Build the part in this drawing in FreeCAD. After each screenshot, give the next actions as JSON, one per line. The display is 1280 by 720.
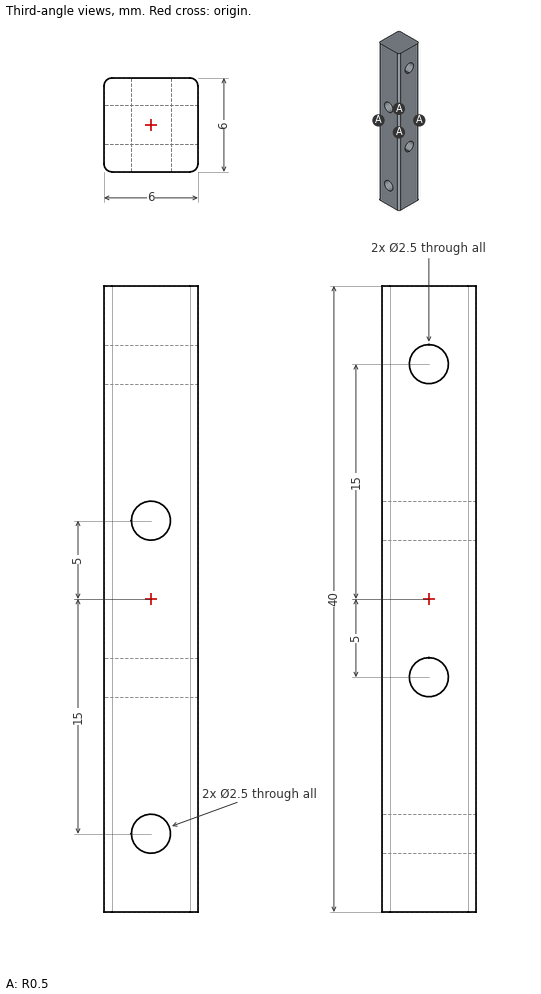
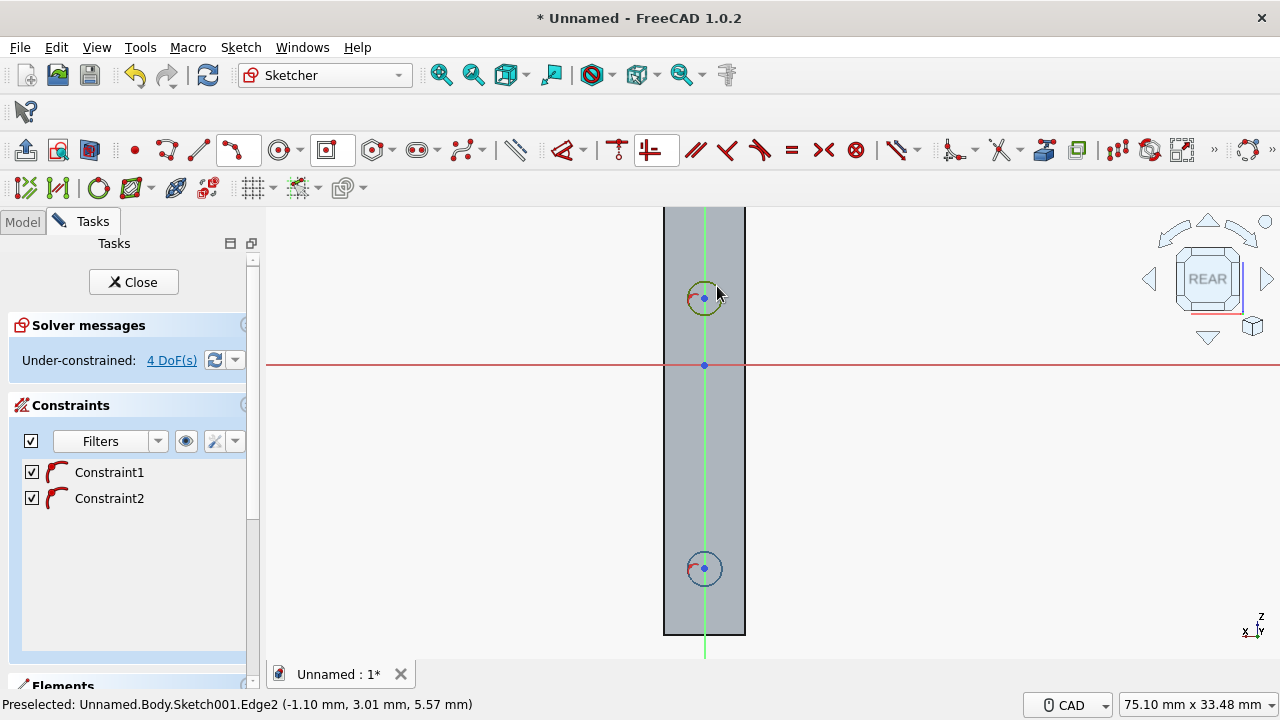
{"action": "left_click", "coordinate": [792, 150]}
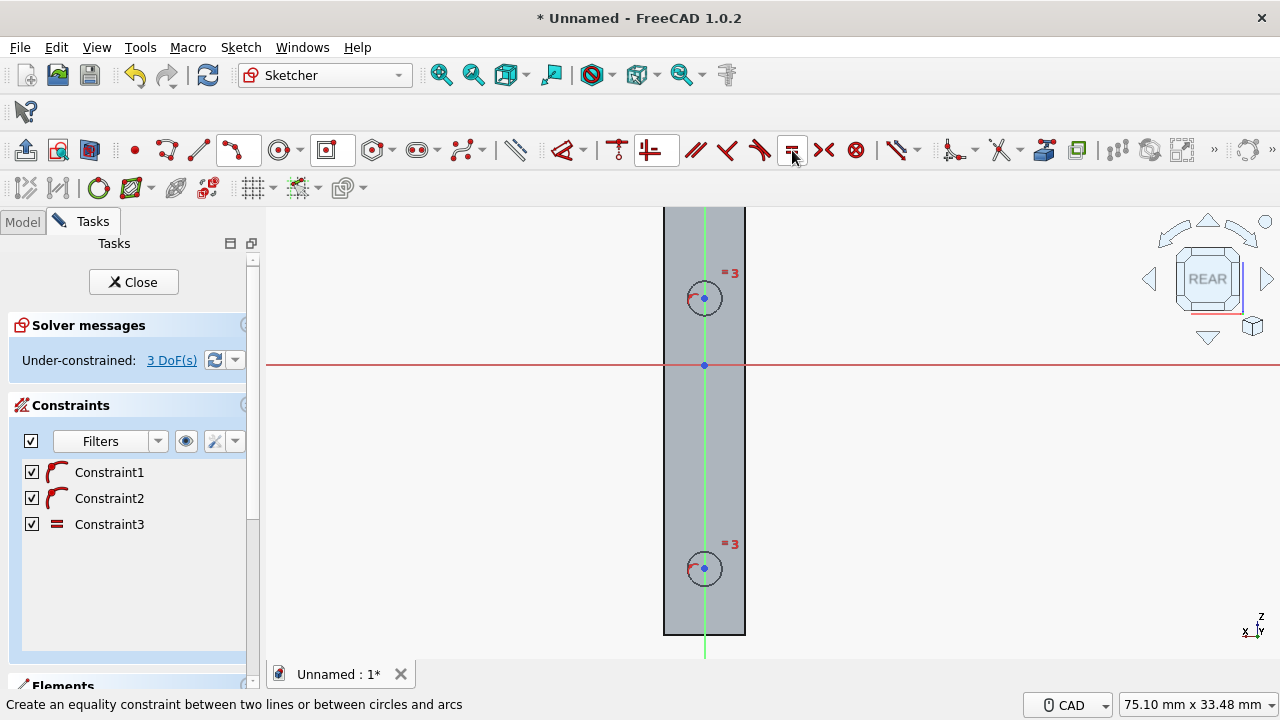
{"action": "left_click", "coordinate": [562, 150]}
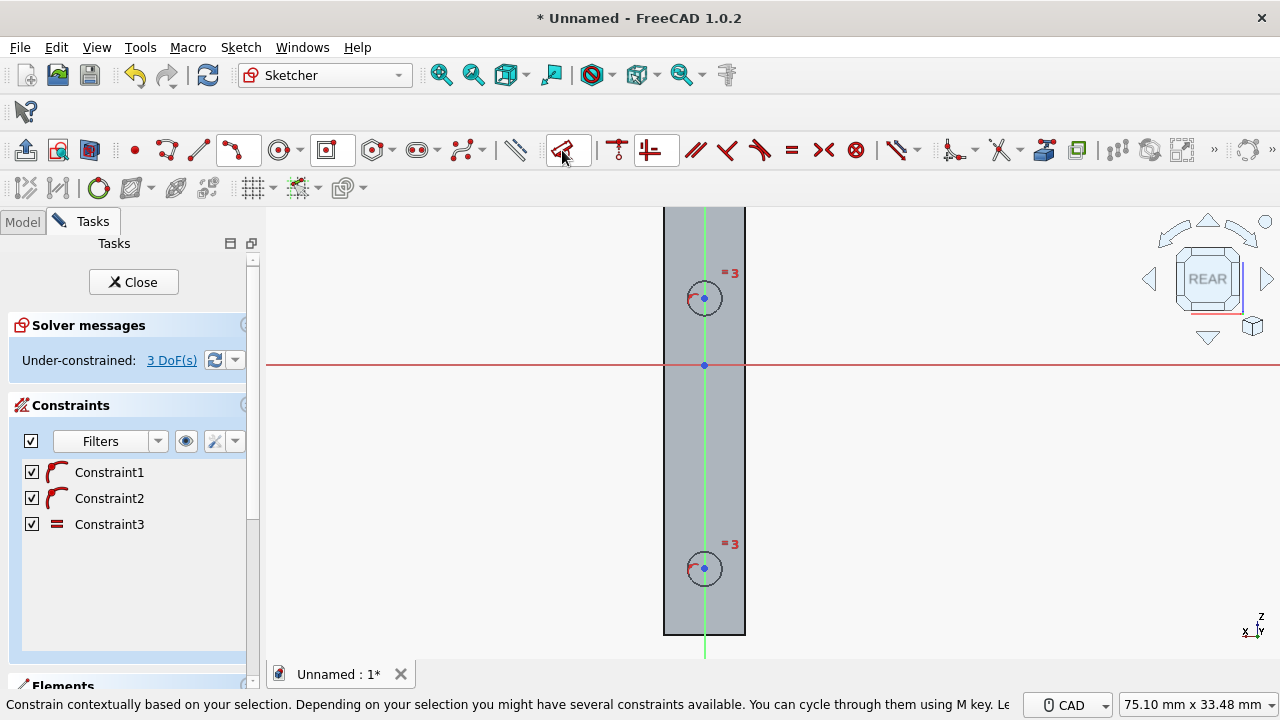
{"action": "left_click", "coordinate": [717, 557]}
{"action": "left_click", "coordinate": [740, 535]}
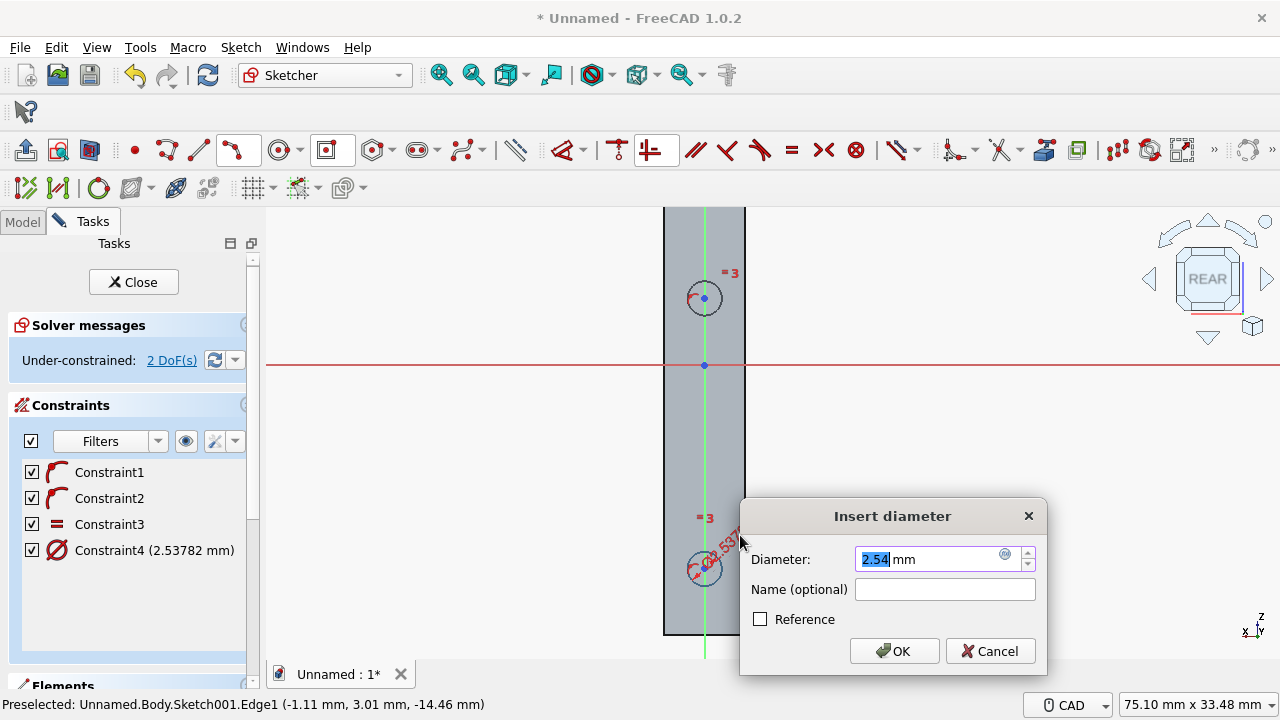
{"action": "type", "text": "2.5"}
{"action": "key", "text": "Return"}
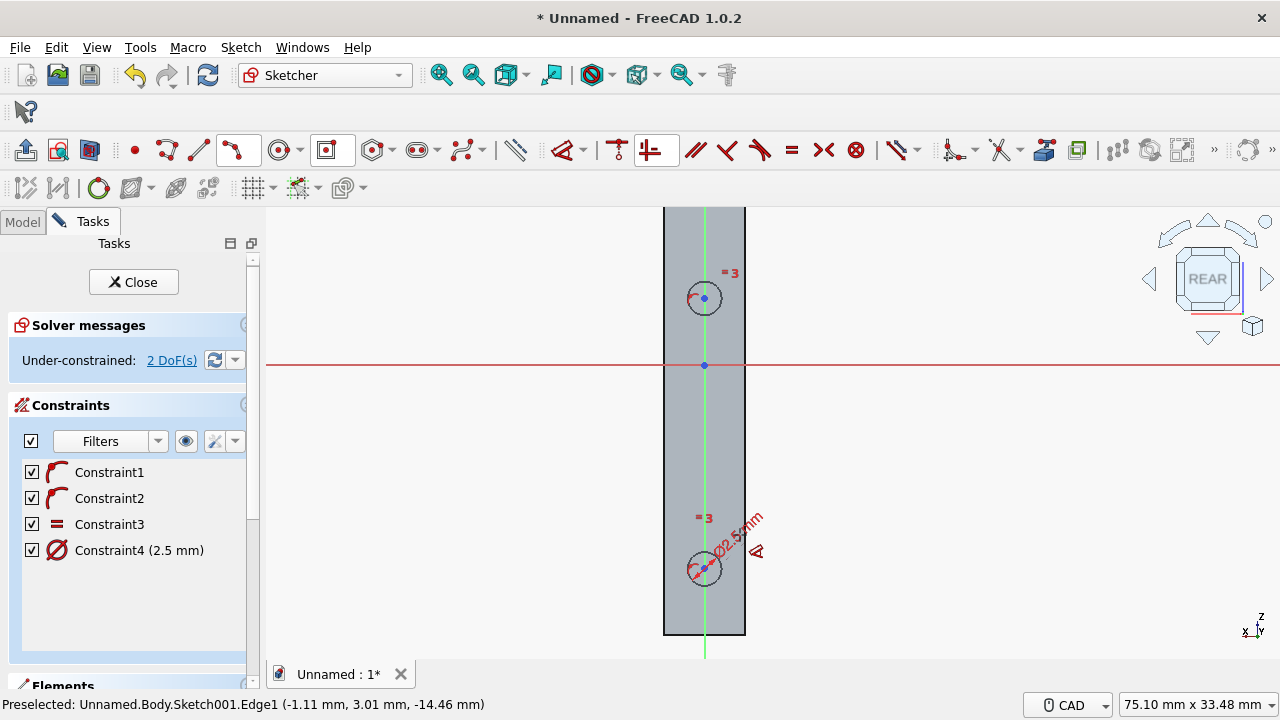
{"action": "left_click", "coordinate": [705, 298]}
{"action": "left_click", "coordinate": [739, 332]}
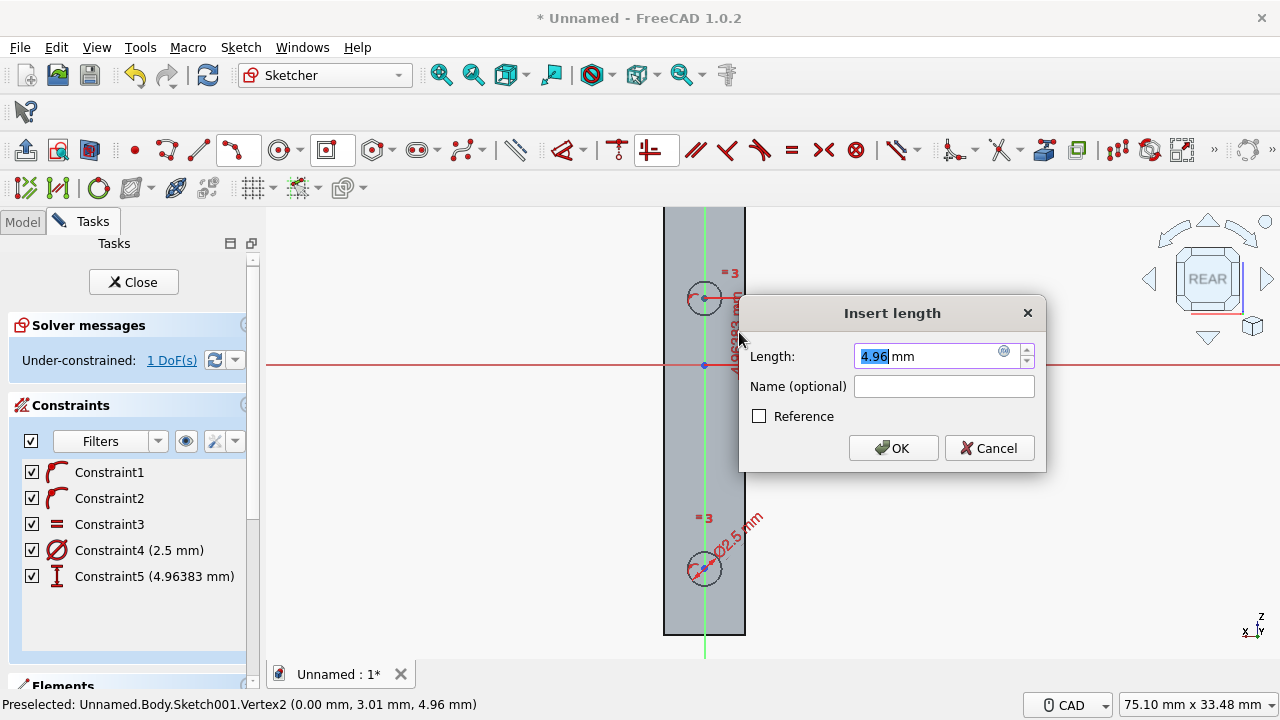
{"action": "type", "text": "5"}
{"action": "key", "text": "Return"}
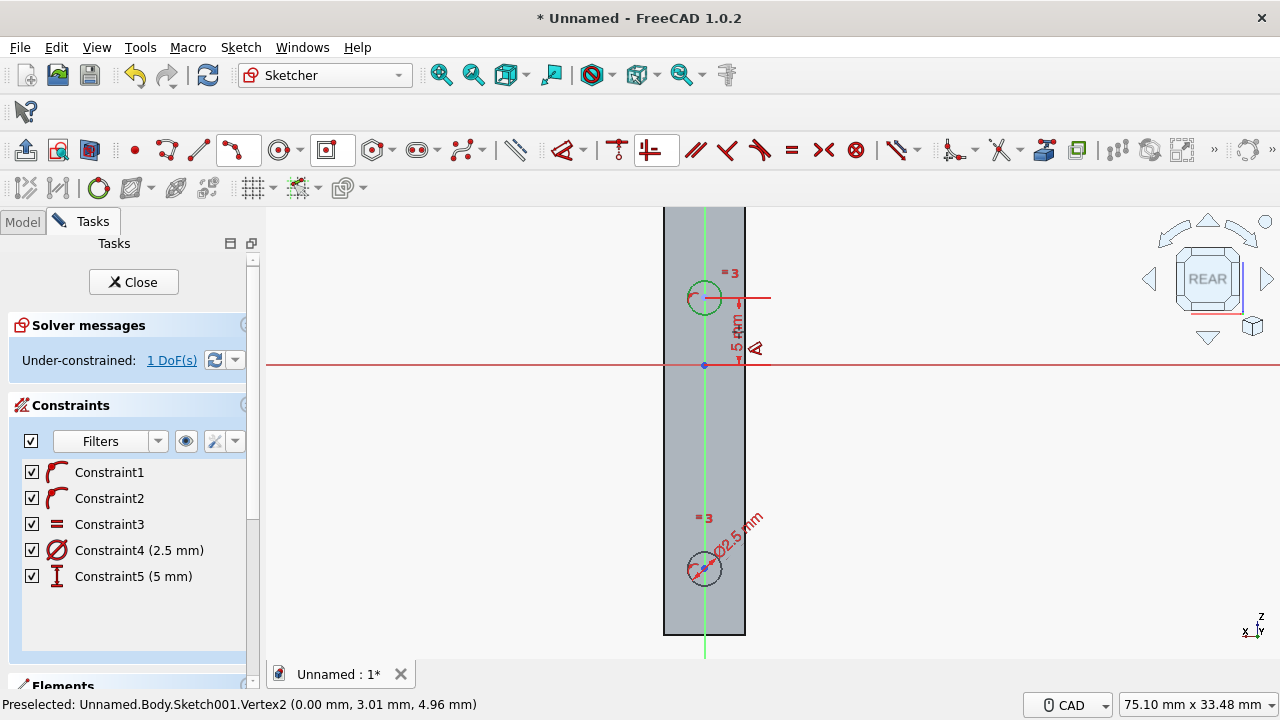
{"action": "left_click", "coordinate": [705, 569]}
{"action": "left_click", "coordinate": [739, 467]}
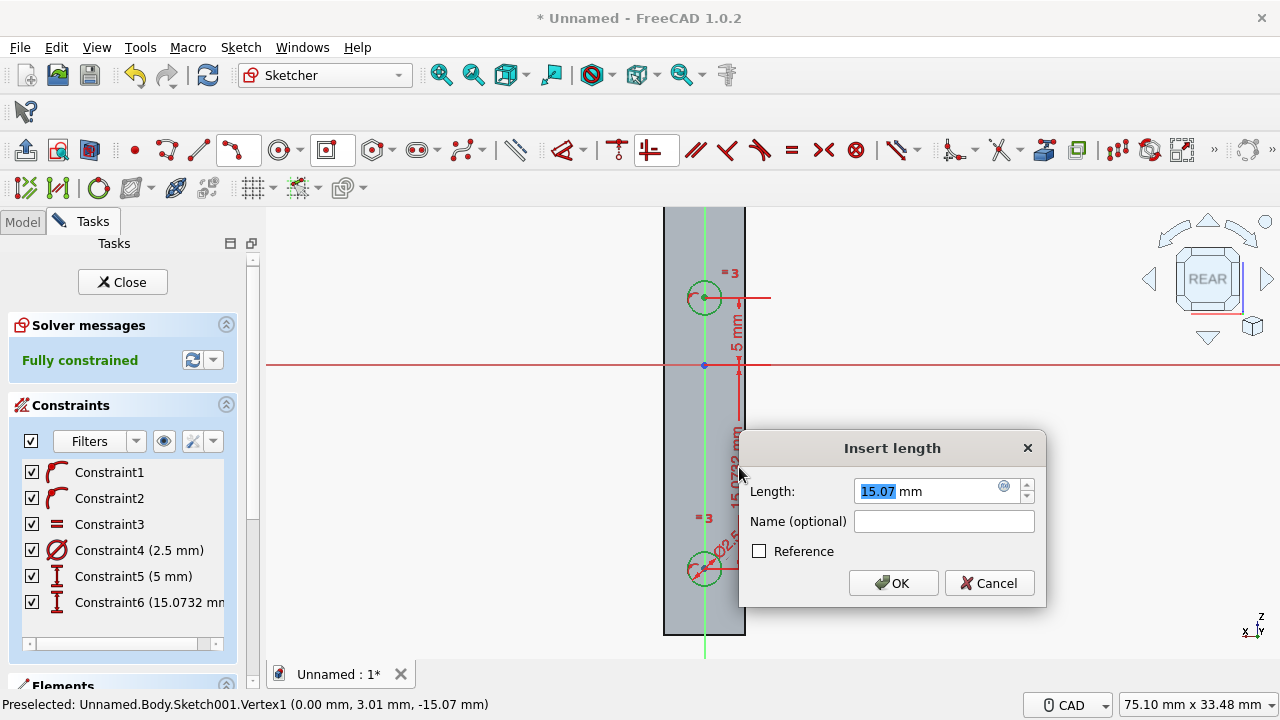
{"action": "type", "text": "15"}
{"action": "key", "text": "Return"}
{"action": "key", "text": "Escape"}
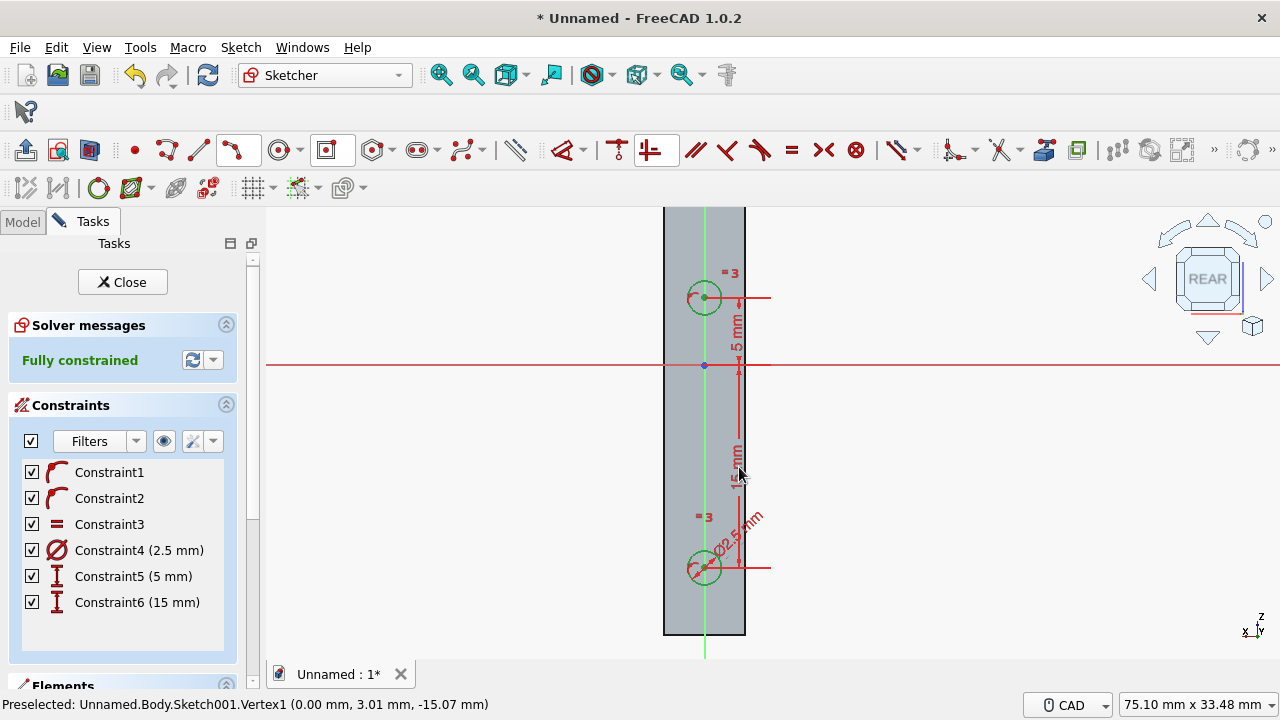
{"action": "left_click", "coordinate": [123, 282]}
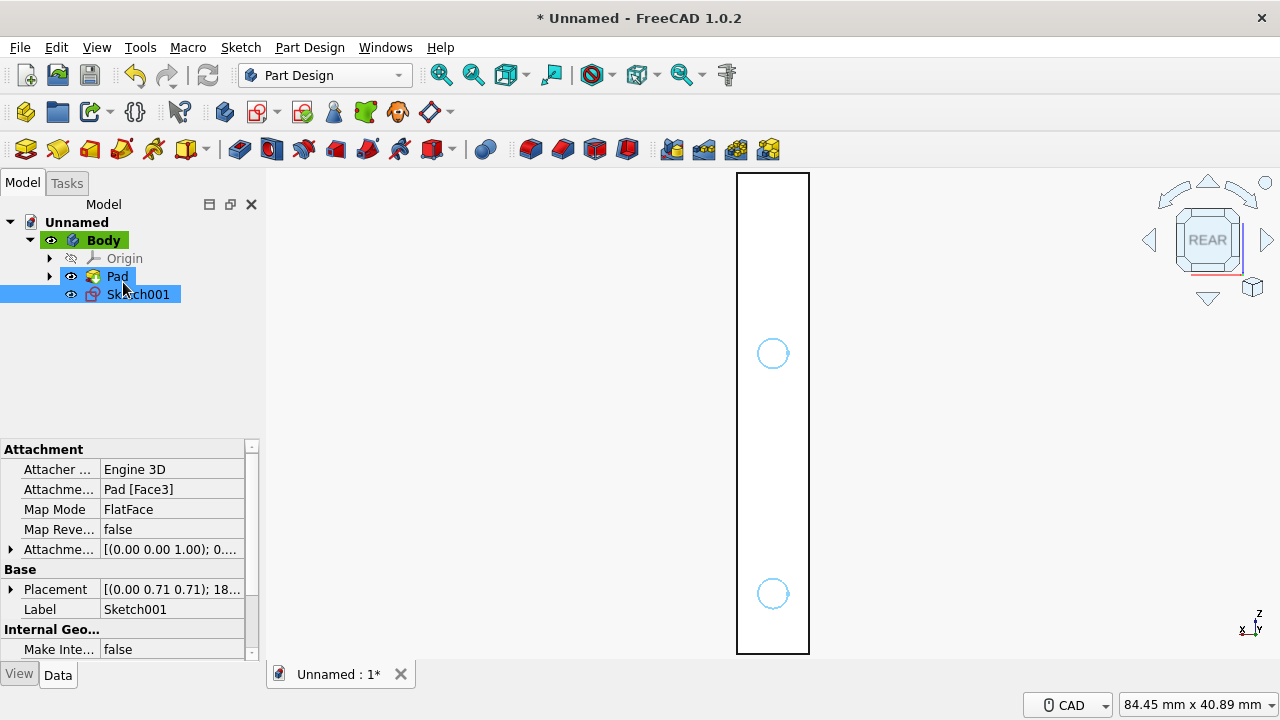
{"action": "left_click", "coordinate": [272, 150]}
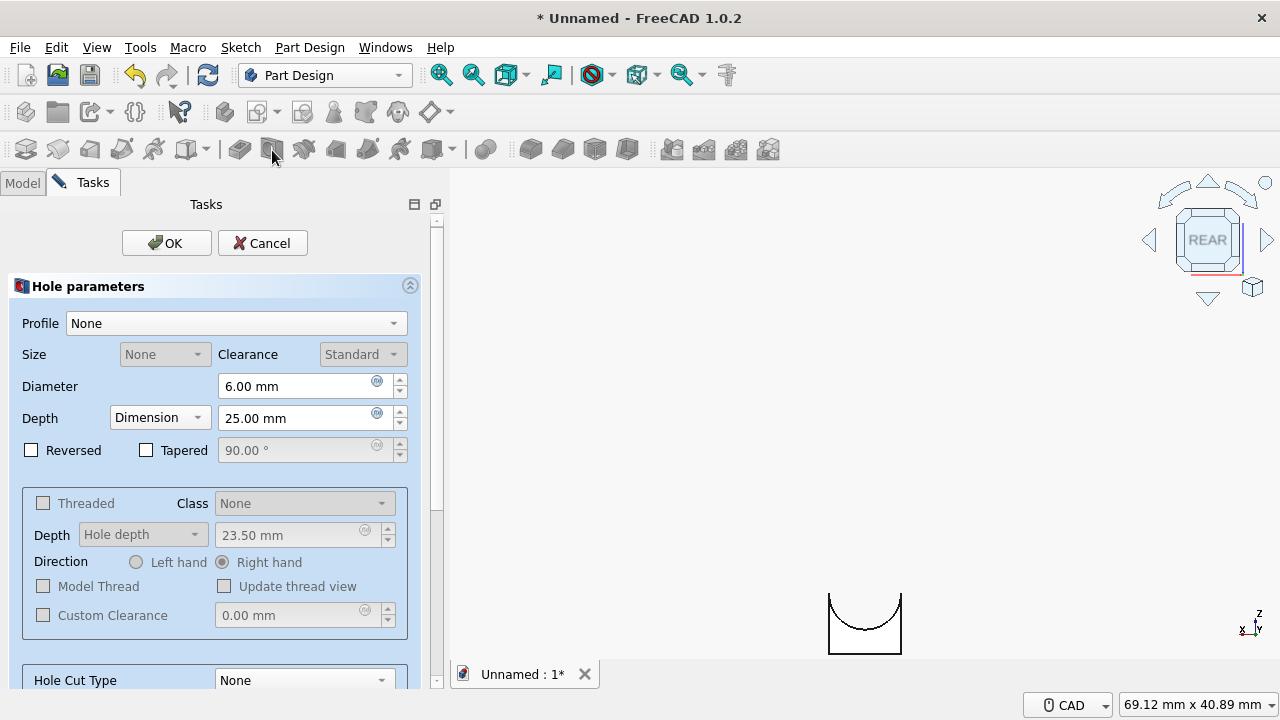
{"action": "triple_click", "coordinate": [305, 386]}